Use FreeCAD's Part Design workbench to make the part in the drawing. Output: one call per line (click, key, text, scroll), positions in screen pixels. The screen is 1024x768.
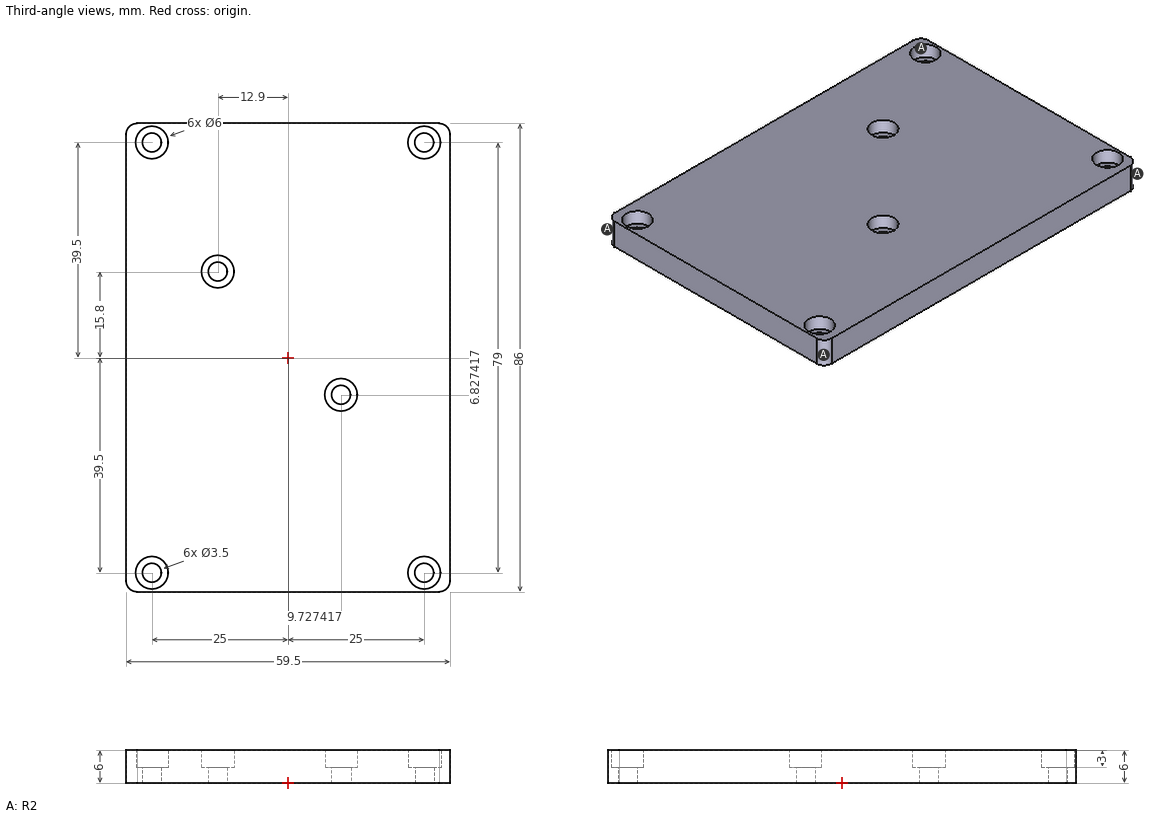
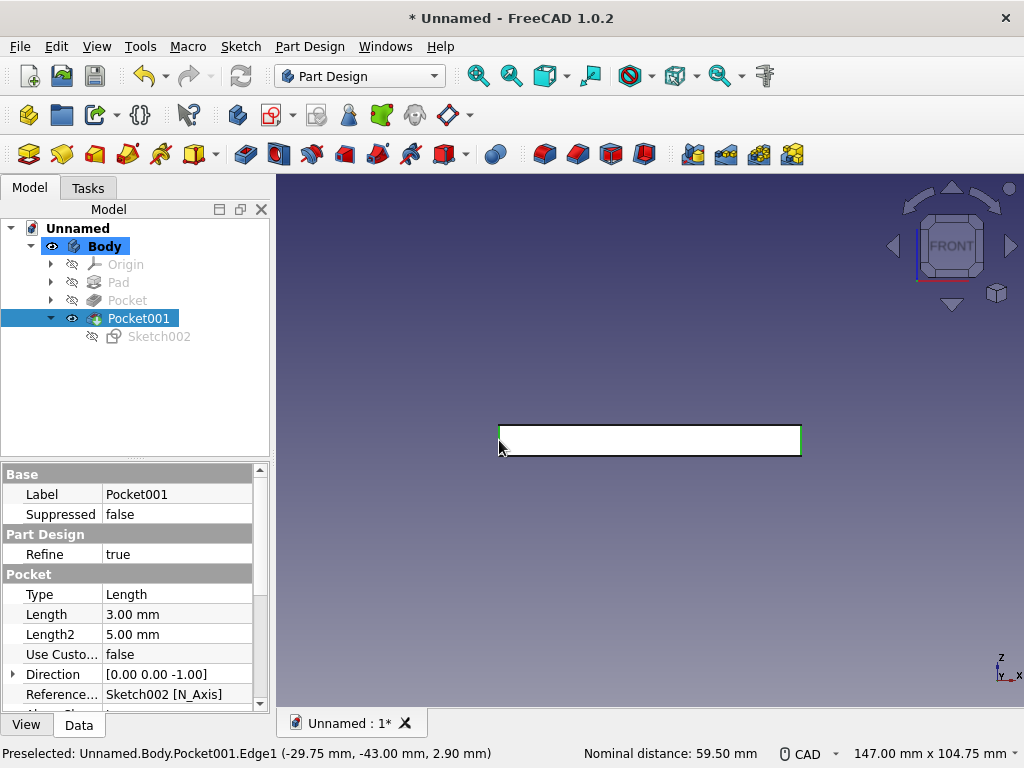
key(3)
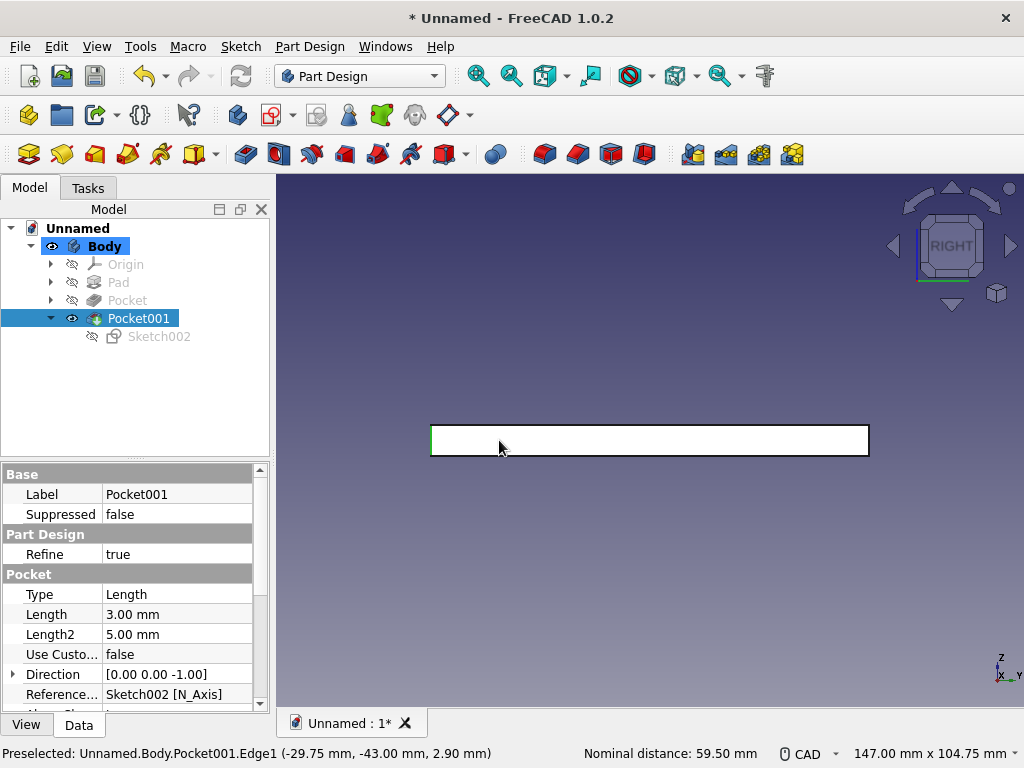
click(869, 439, ctrl)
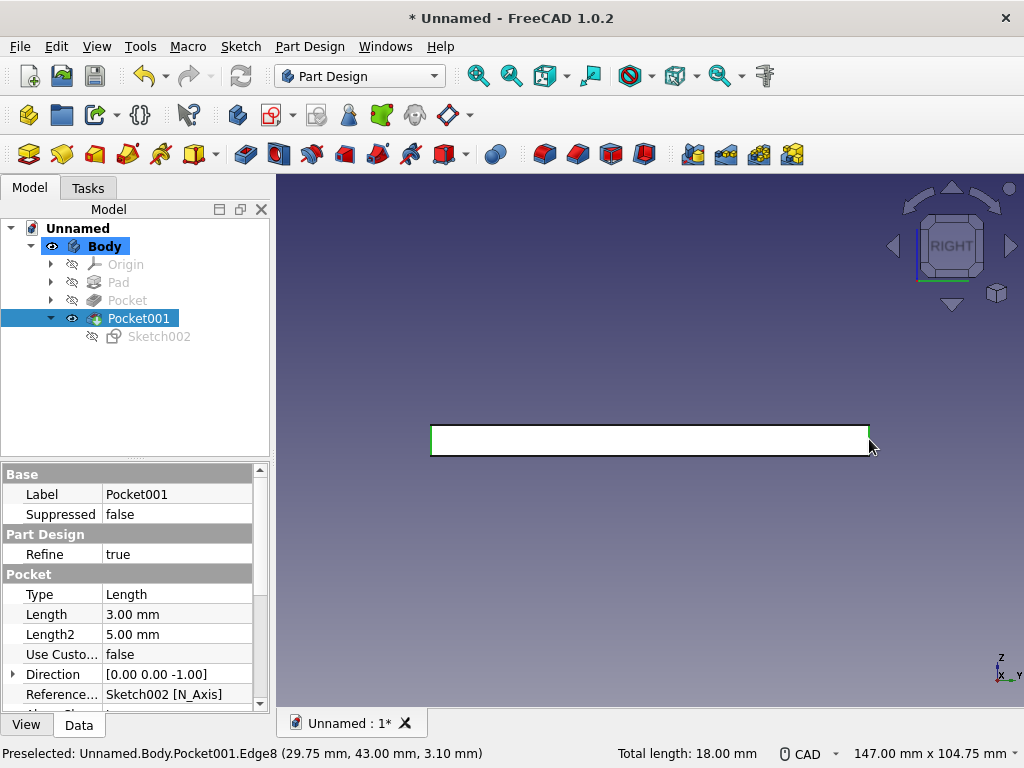
key(5)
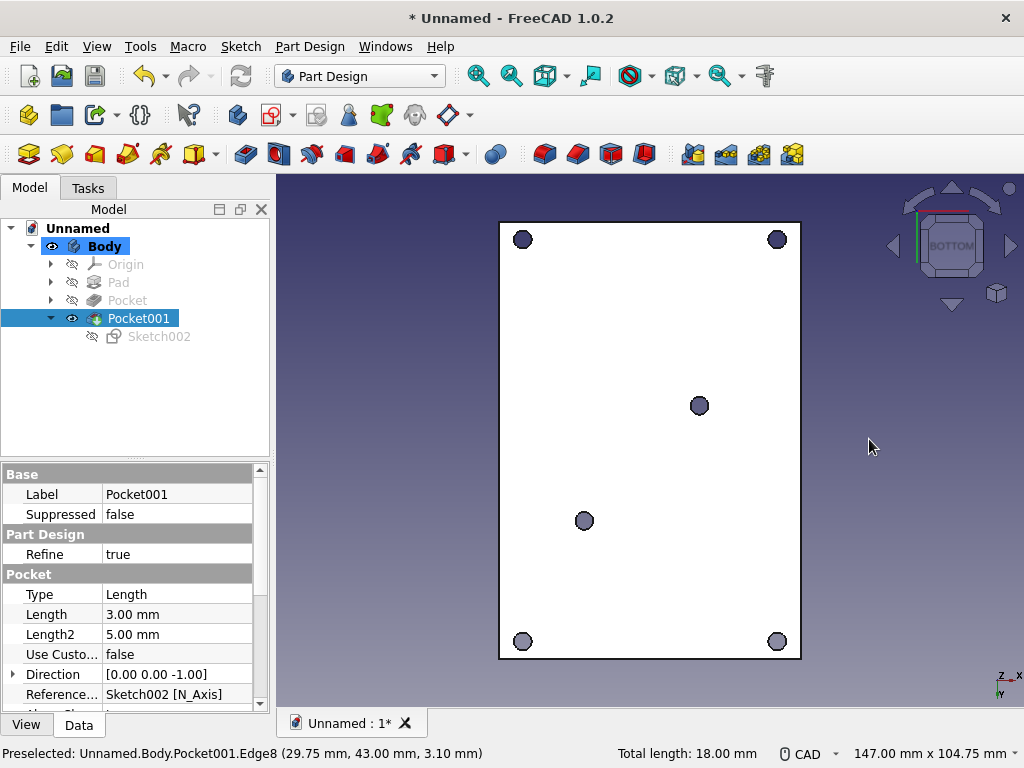
key(4)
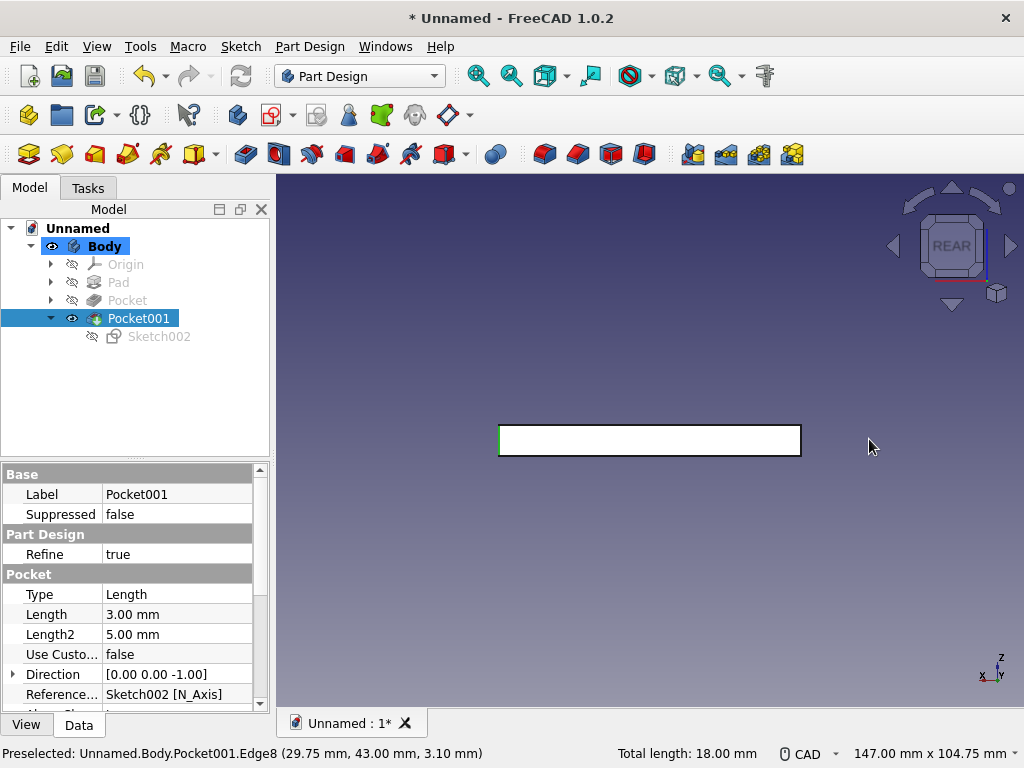
key(v)
key(f)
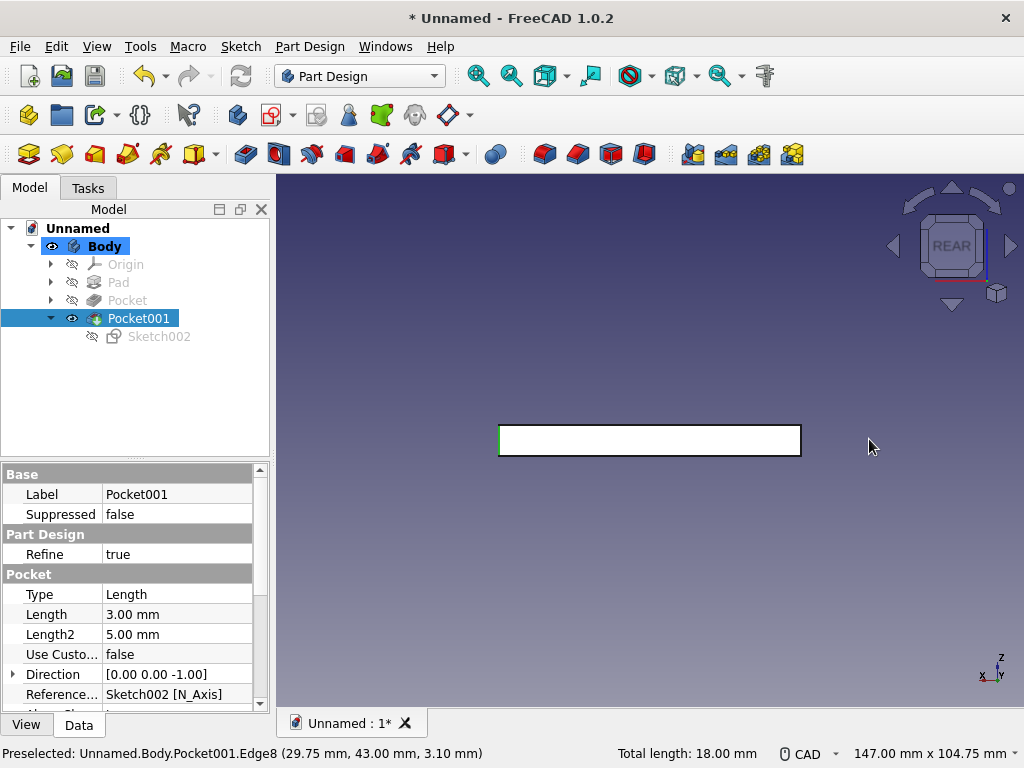
click(801, 440, ctrl)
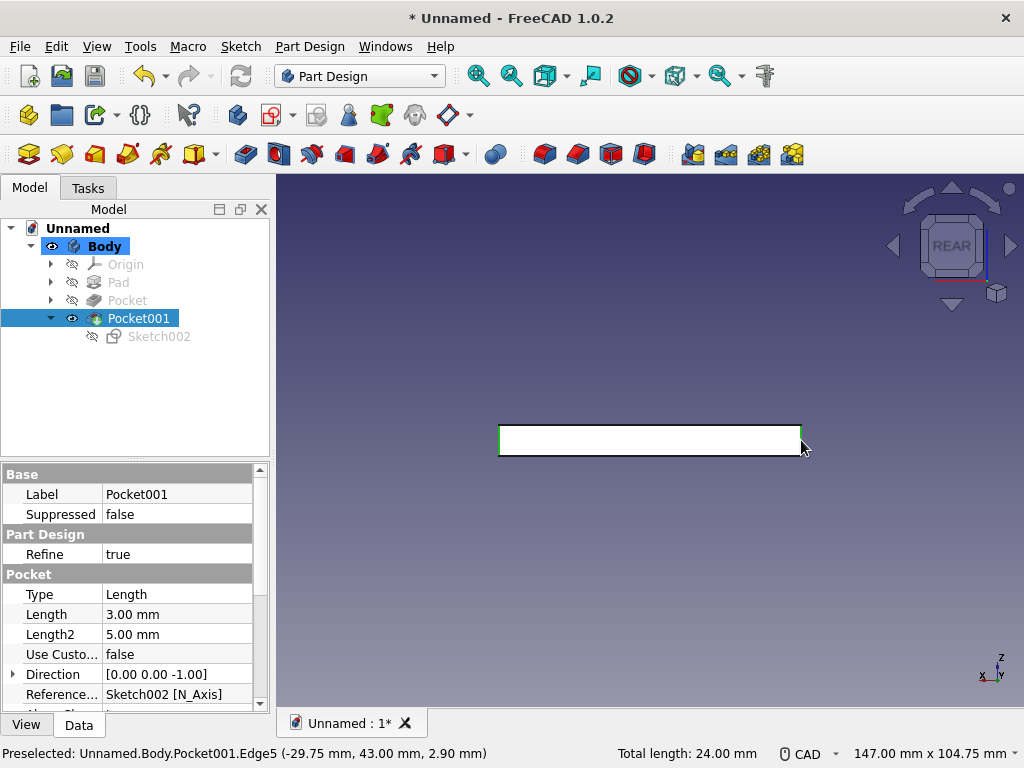
click(545, 154)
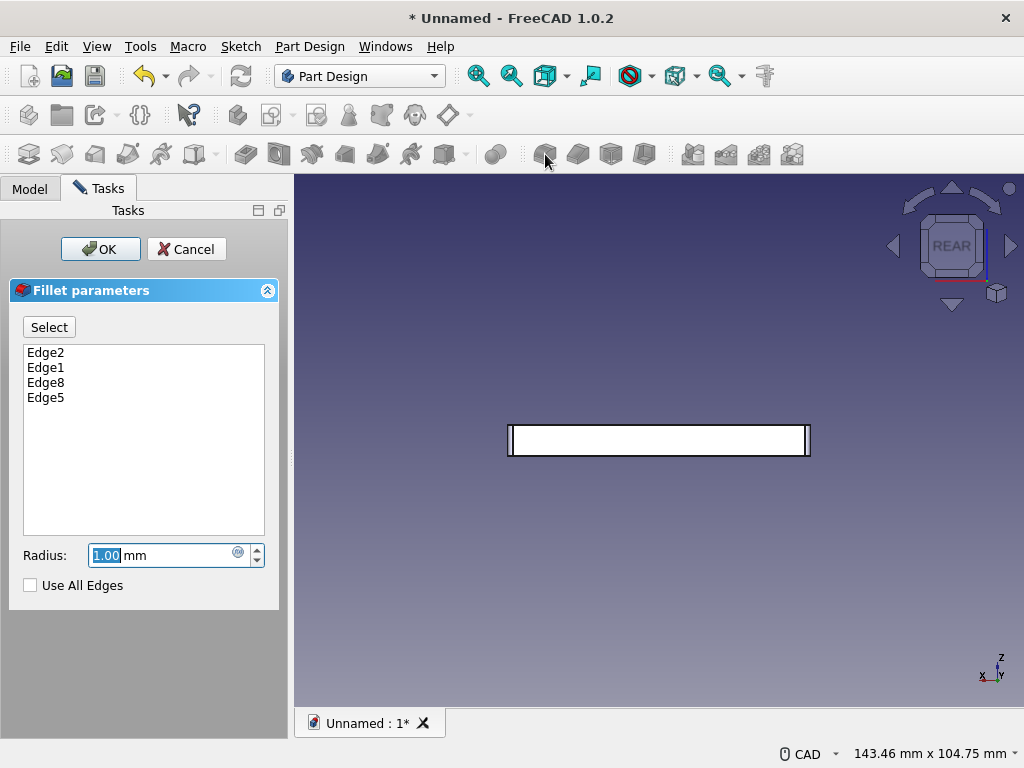
text(2)
key(Tab)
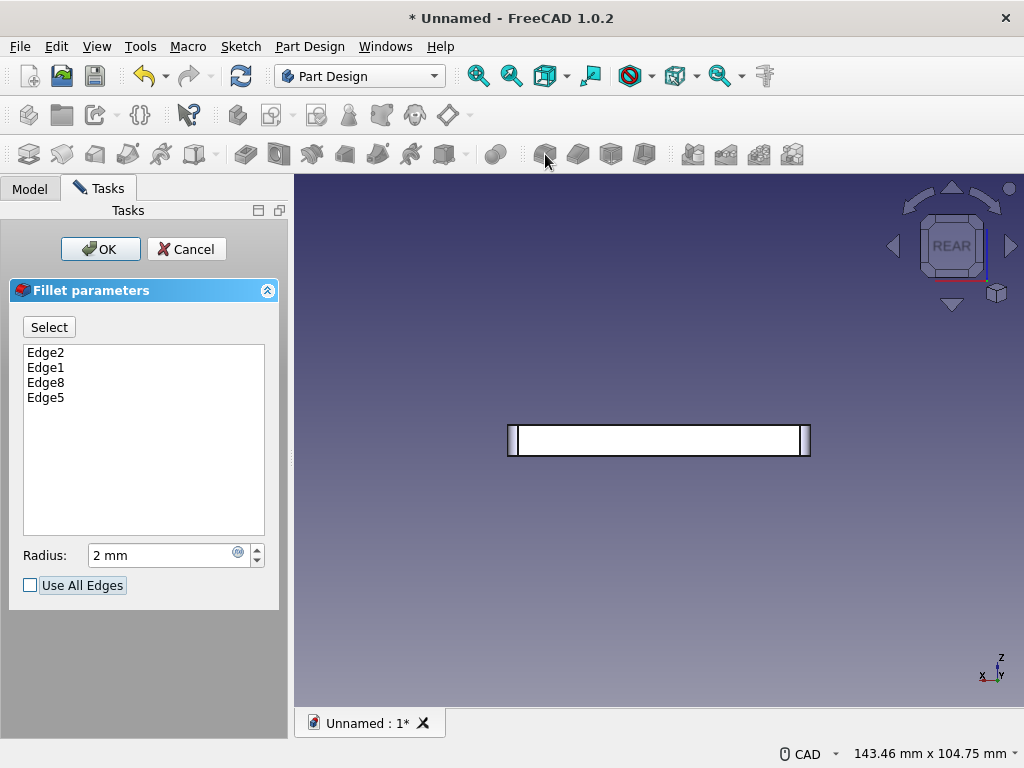
click(101, 249)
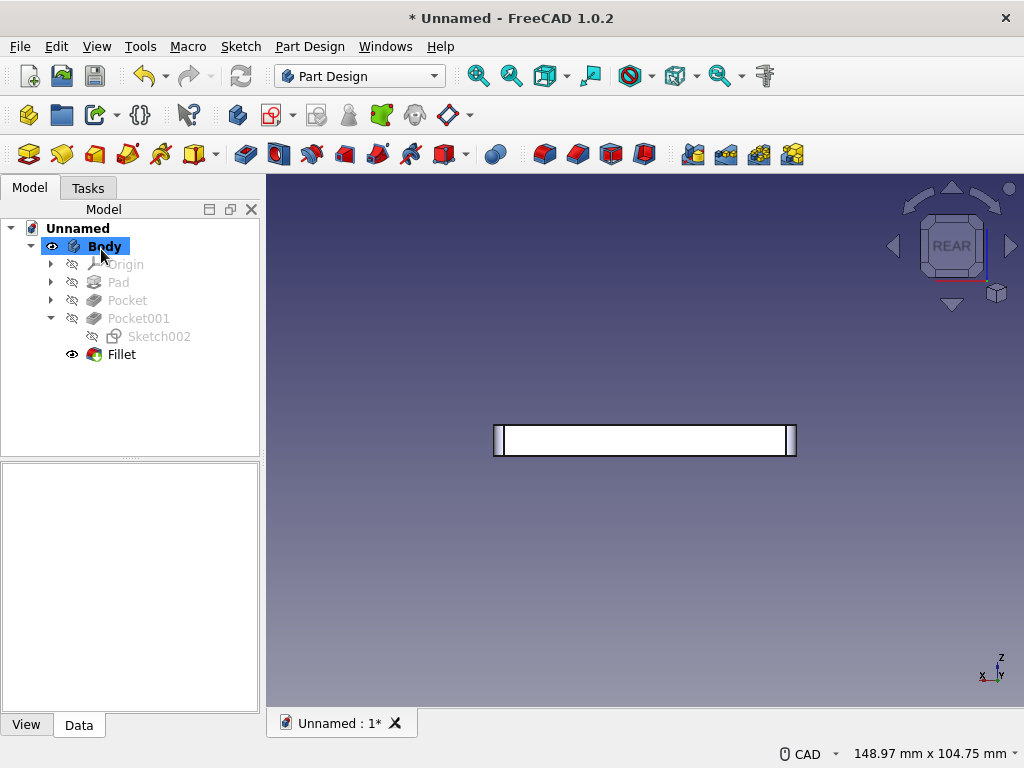
key(0)